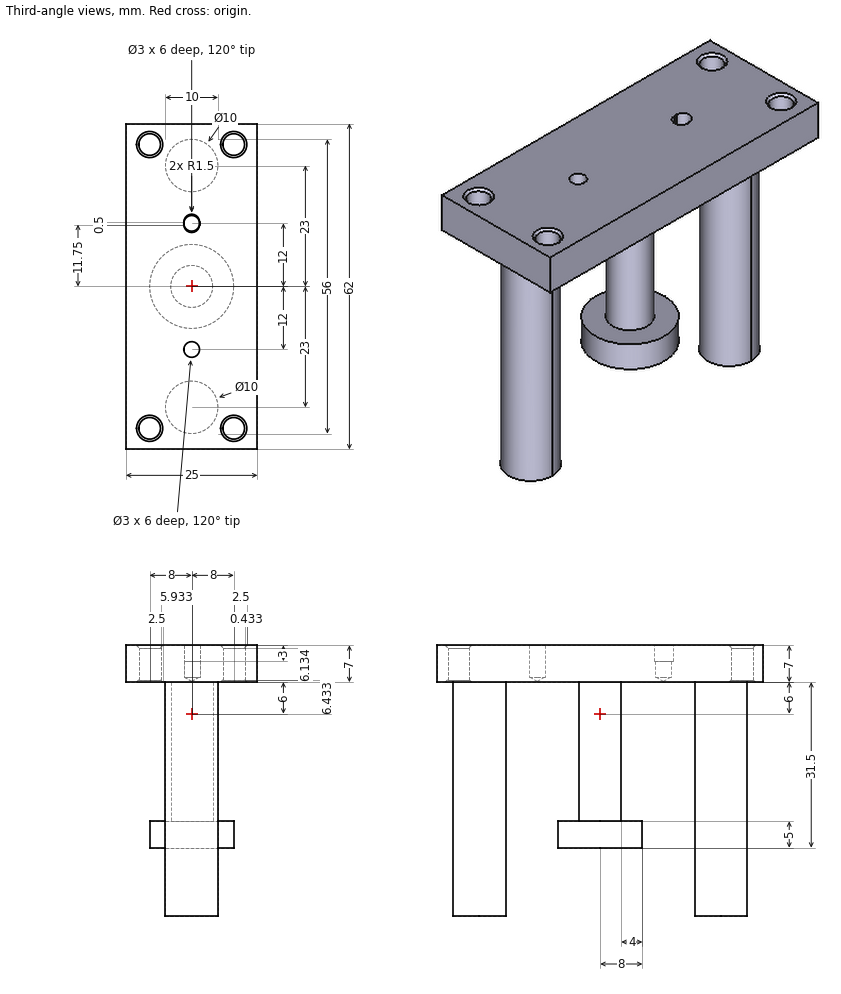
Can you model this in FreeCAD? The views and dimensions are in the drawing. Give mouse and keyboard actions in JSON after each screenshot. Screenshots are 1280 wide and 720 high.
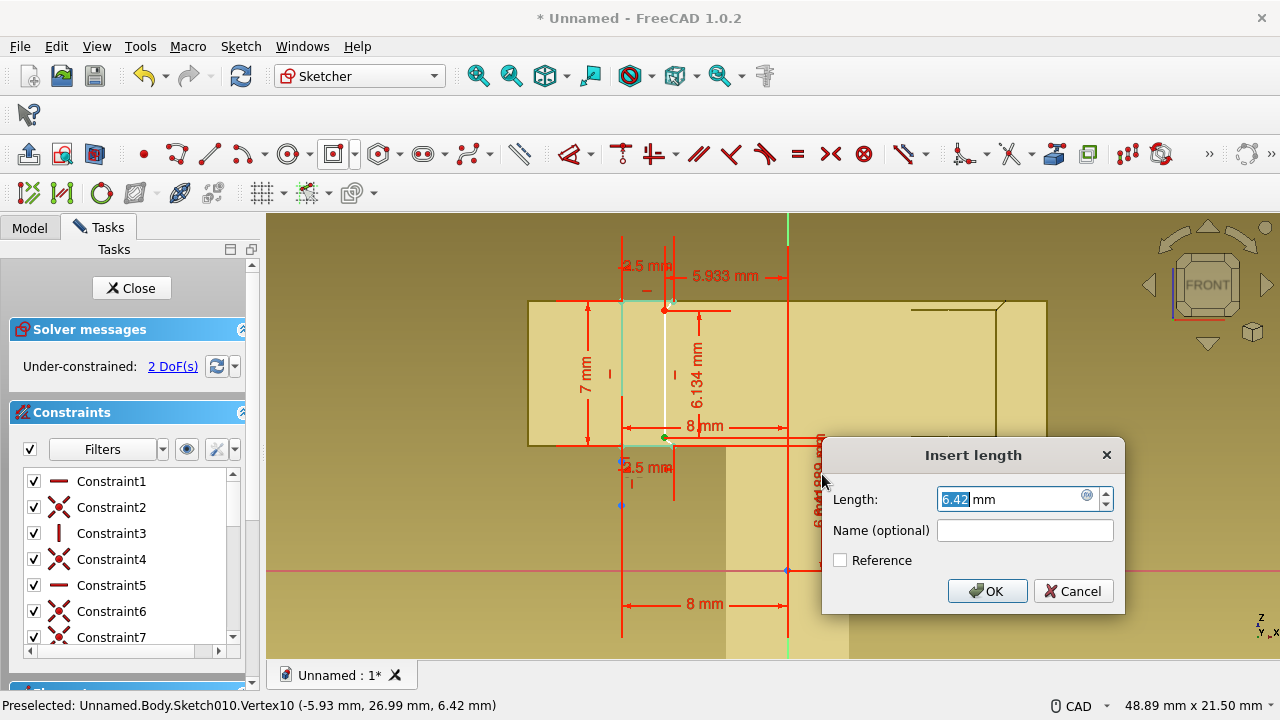
{"action": "type", "text": "6.433"}
{"action": "key", "text": "Return"}
{"action": "key", "text": "Escape"}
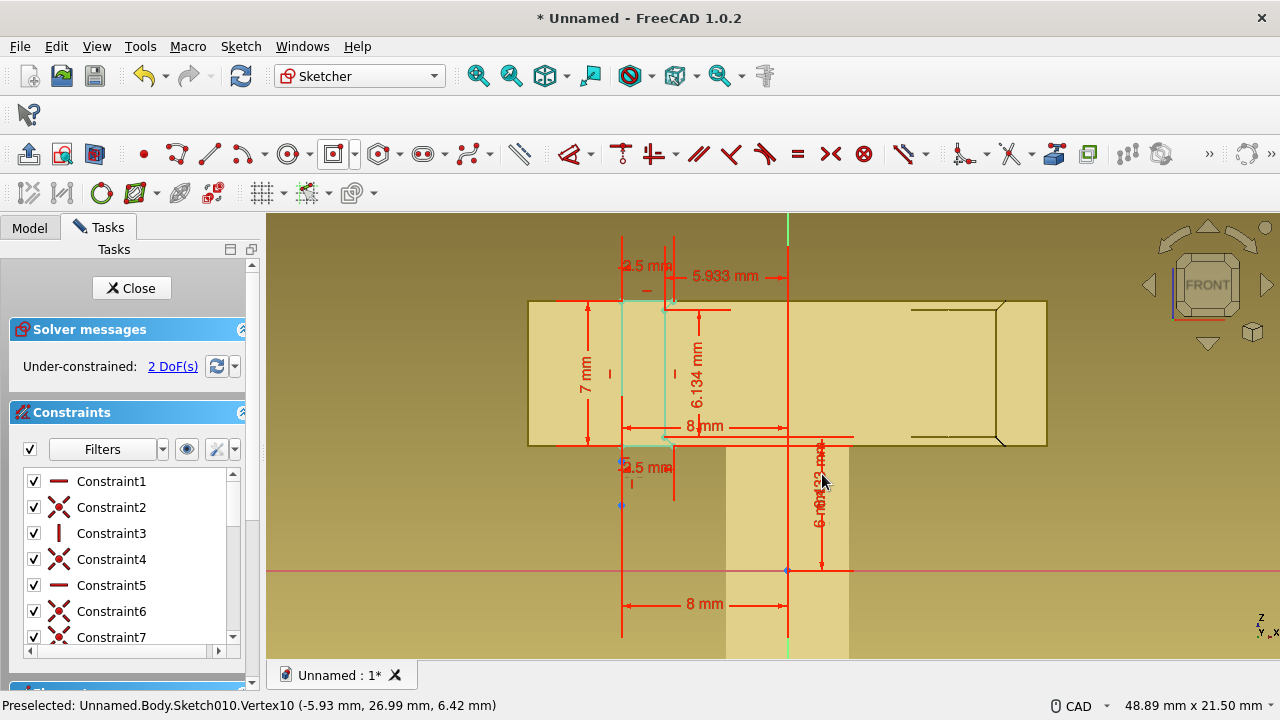
{"action": "left_click", "coordinate": [132, 288]}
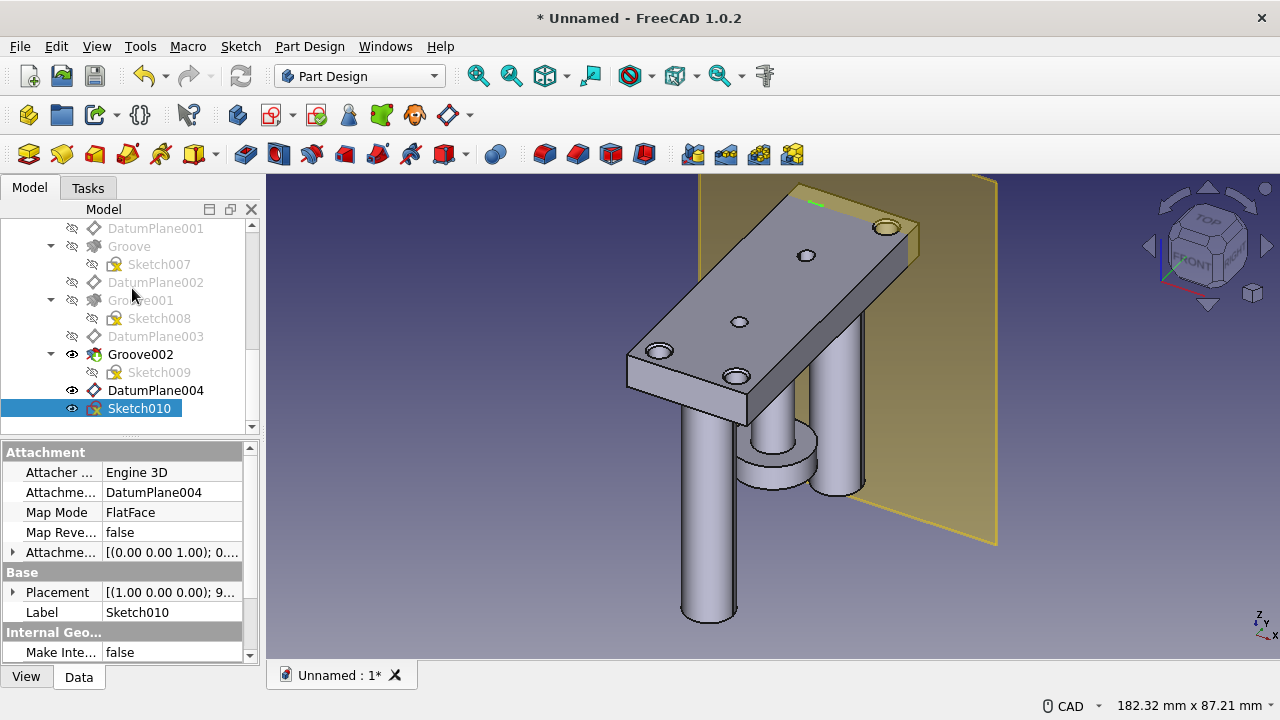
{"action": "left_click", "coordinate": [312, 154]}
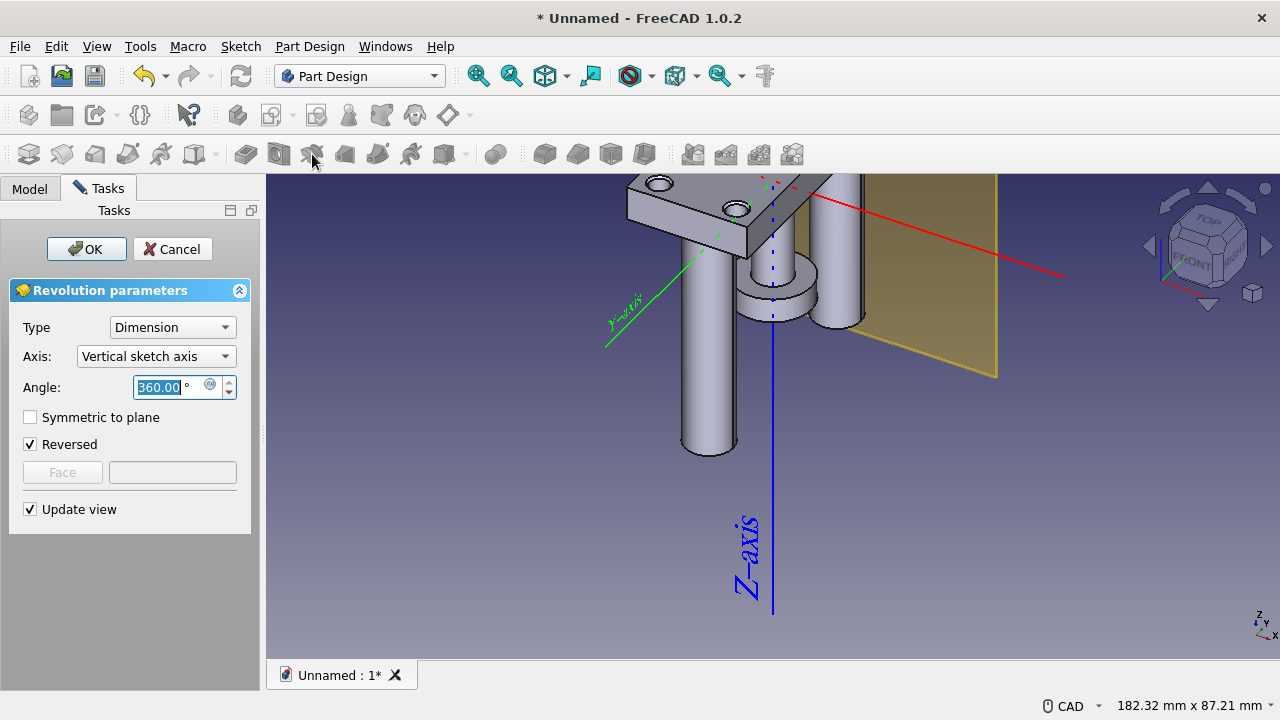
{"action": "left_click", "coordinate": [157, 356]}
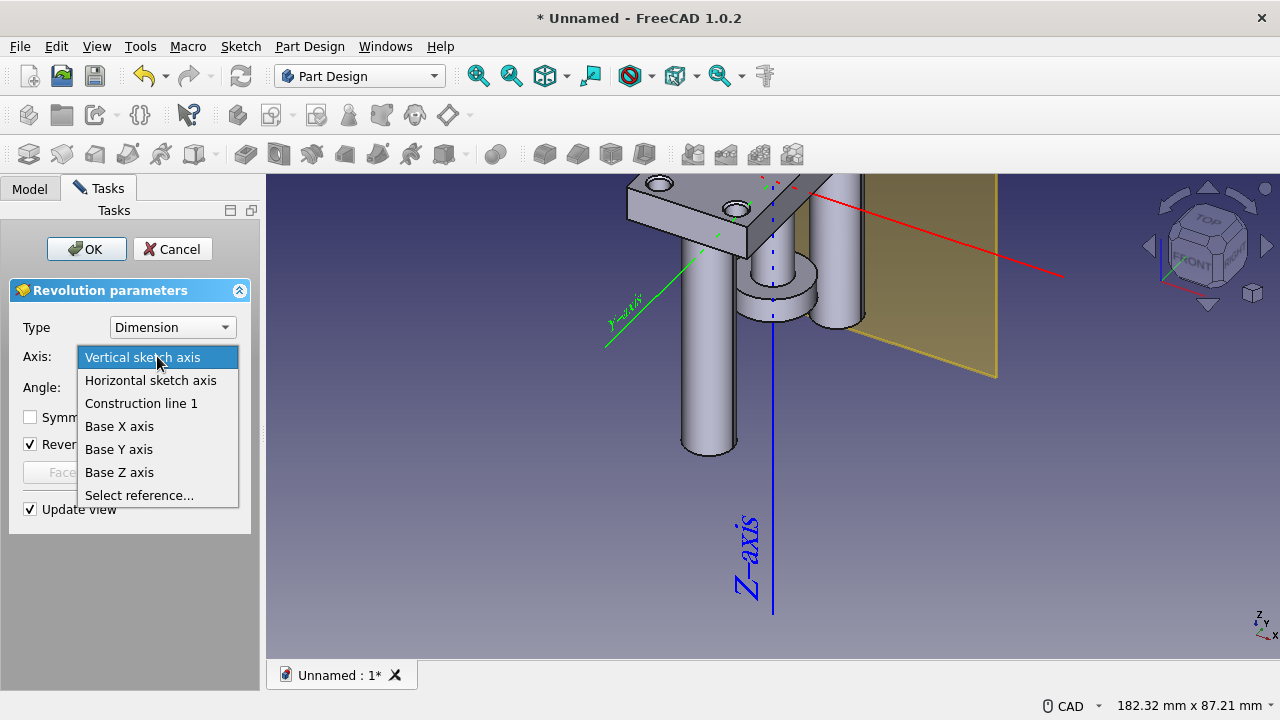
{"action": "left_click", "coordinate": [156, 404]}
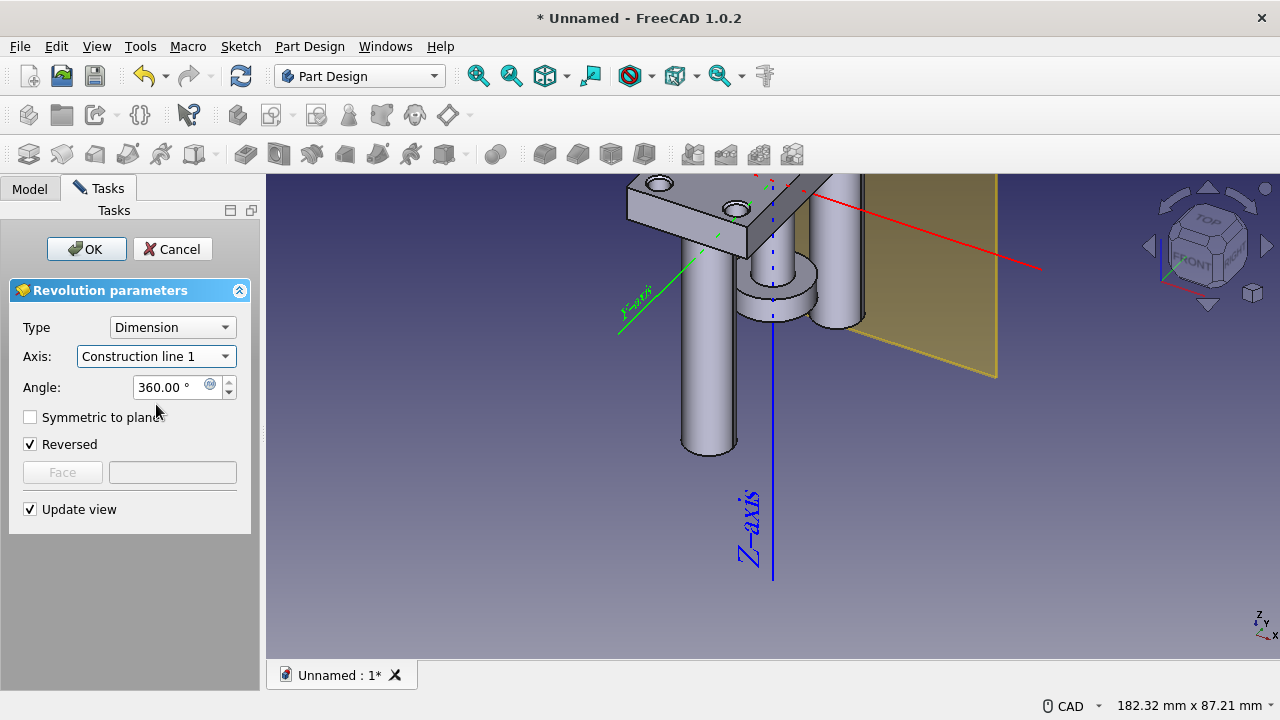
{"action": "left_click", "coordinate": [87, 249]}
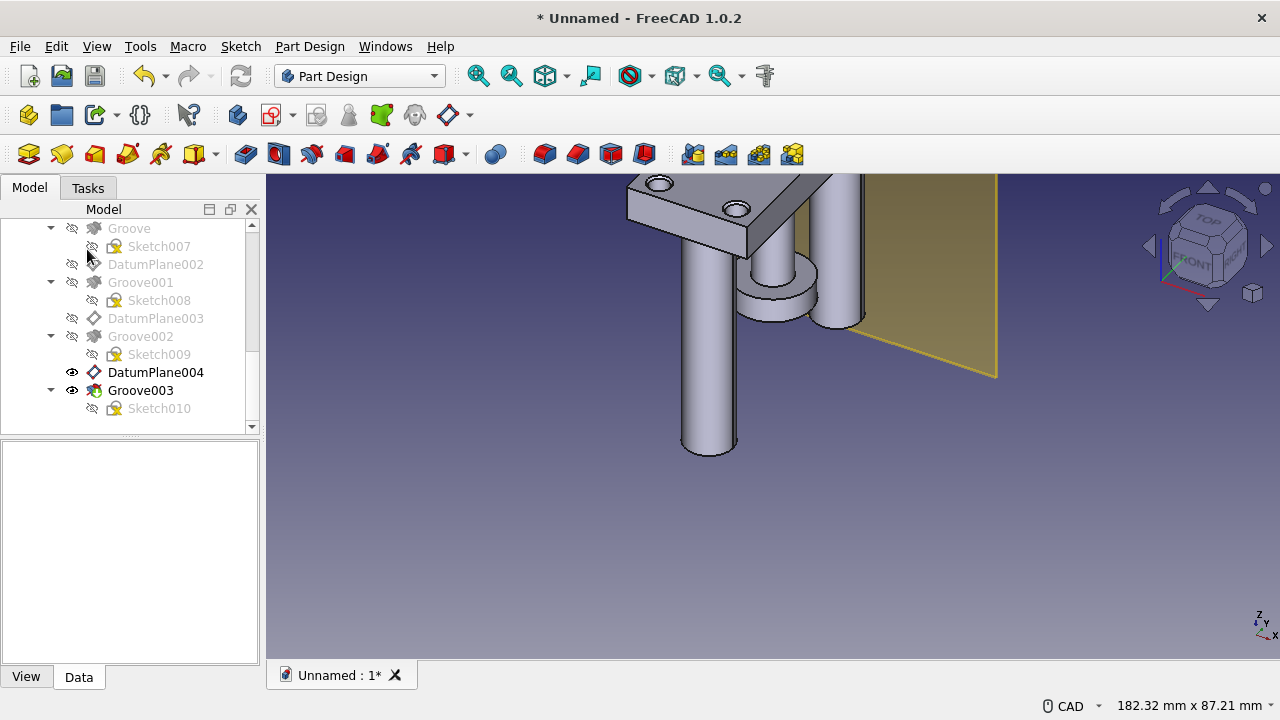
{"action": "left_click", "coordinate": [117, 372]}
{"action": "key", "text": "space"}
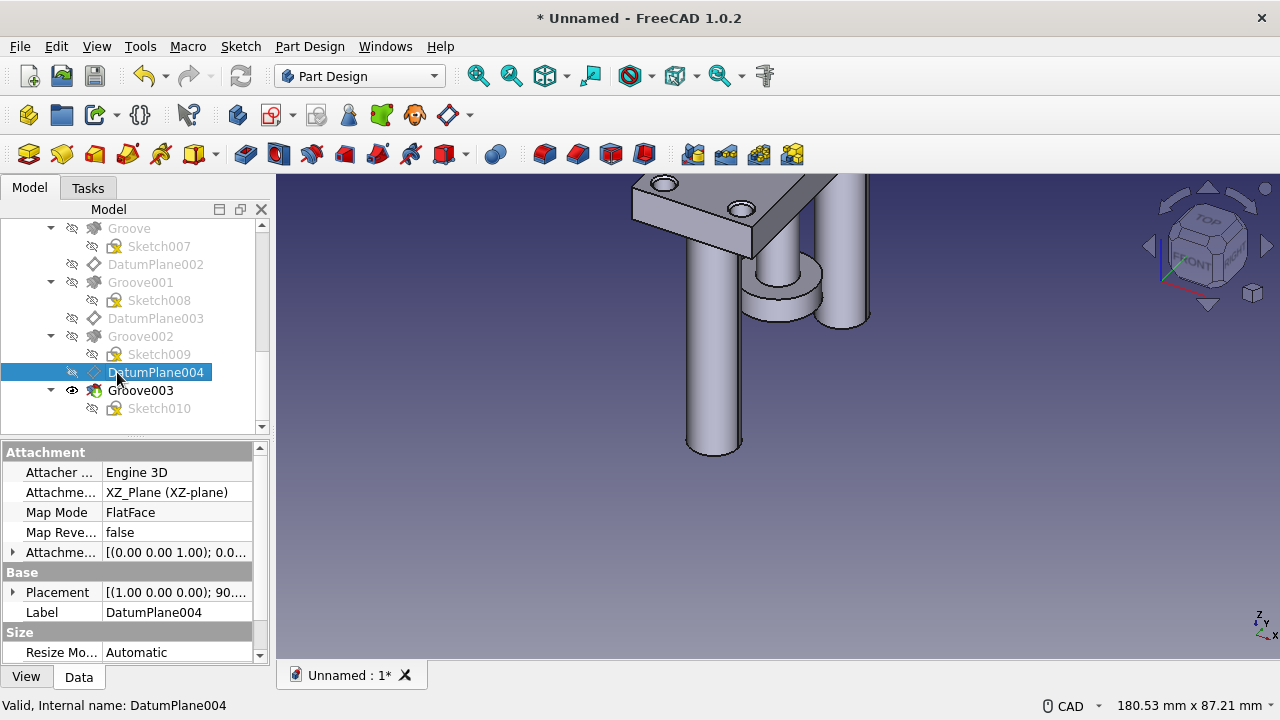
{"action": "left_click", "coordinate": [479, 76]}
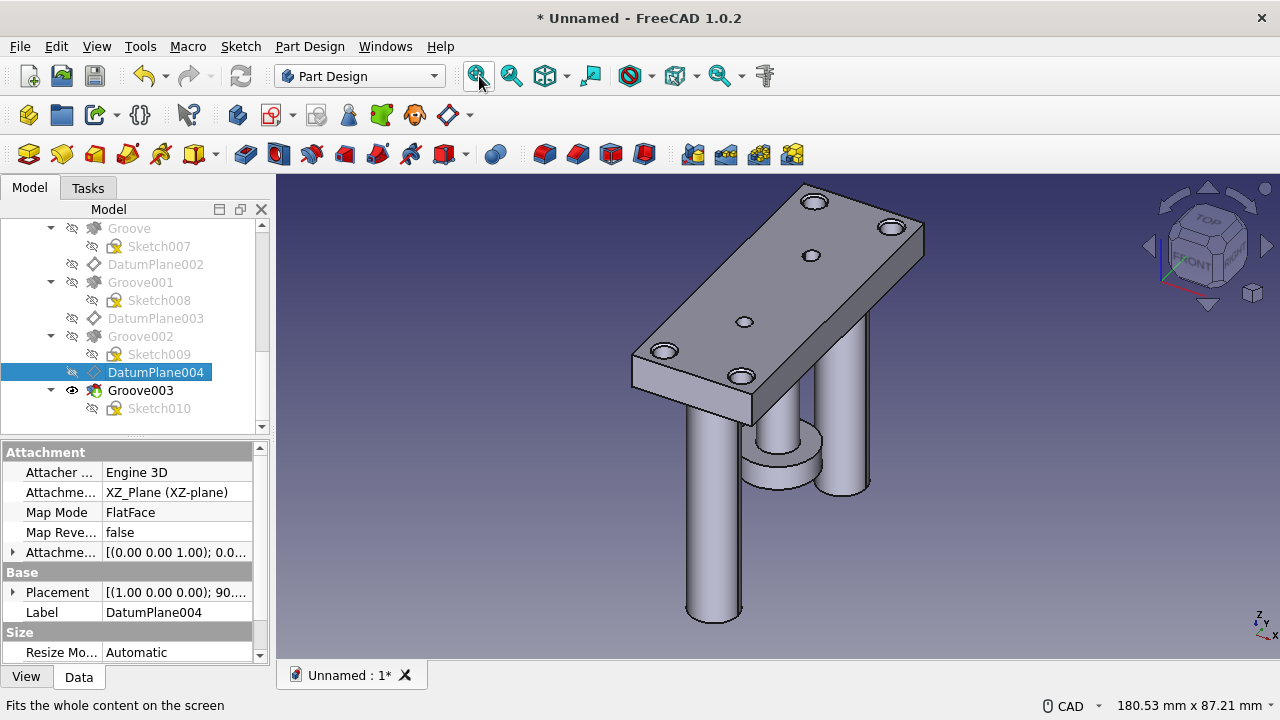
{"action": "key", "text": "5"}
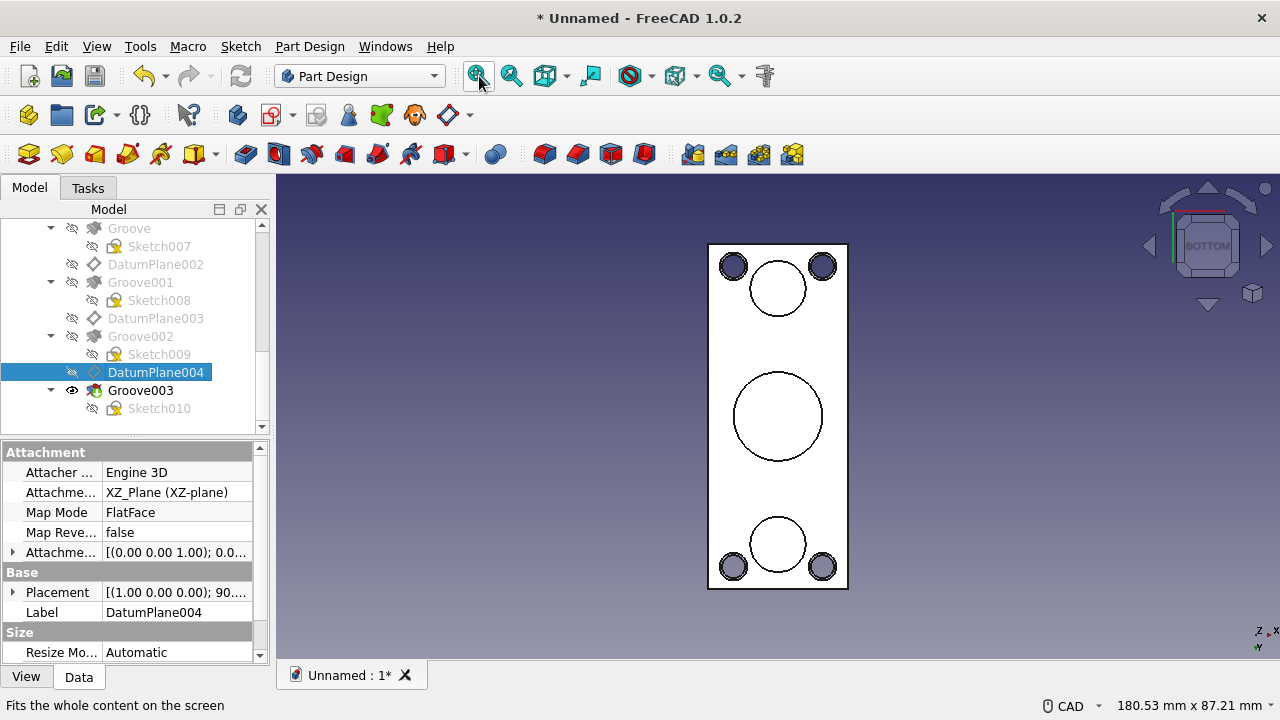
{"action": "left_click", "coordinate": [778, 543]}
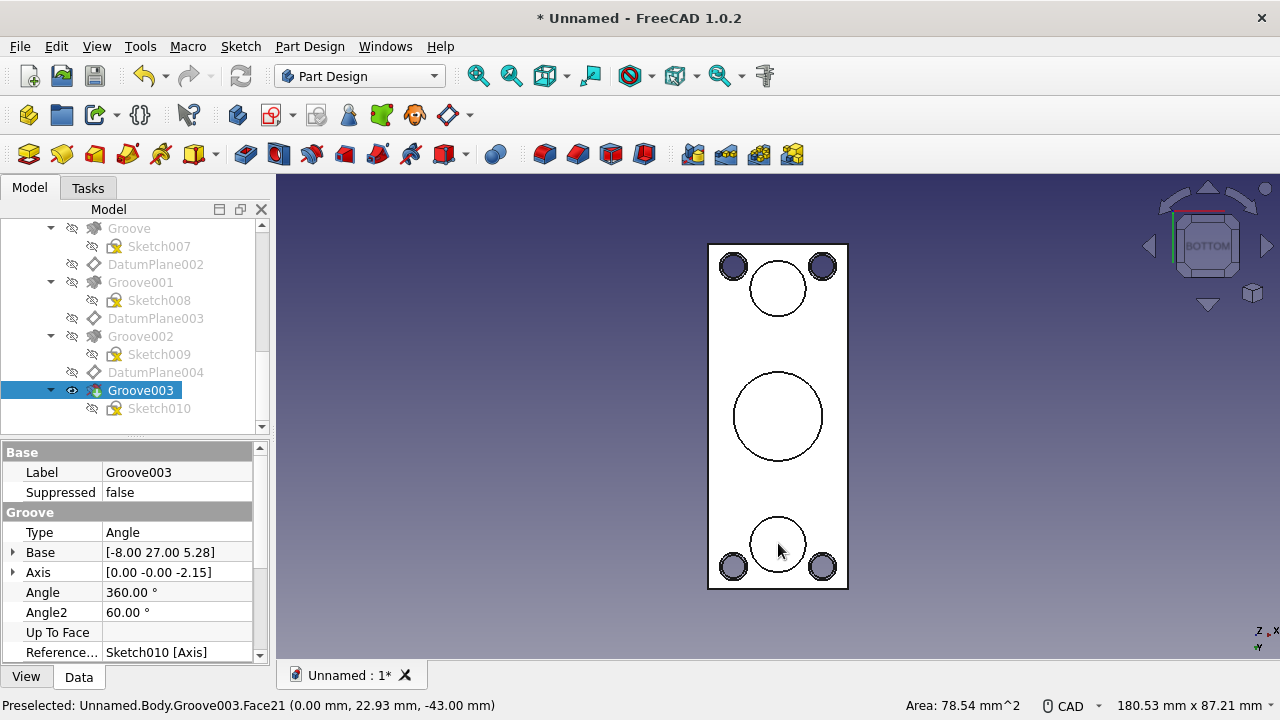
{"action": "left_click", "coordinate": [270, 116]}